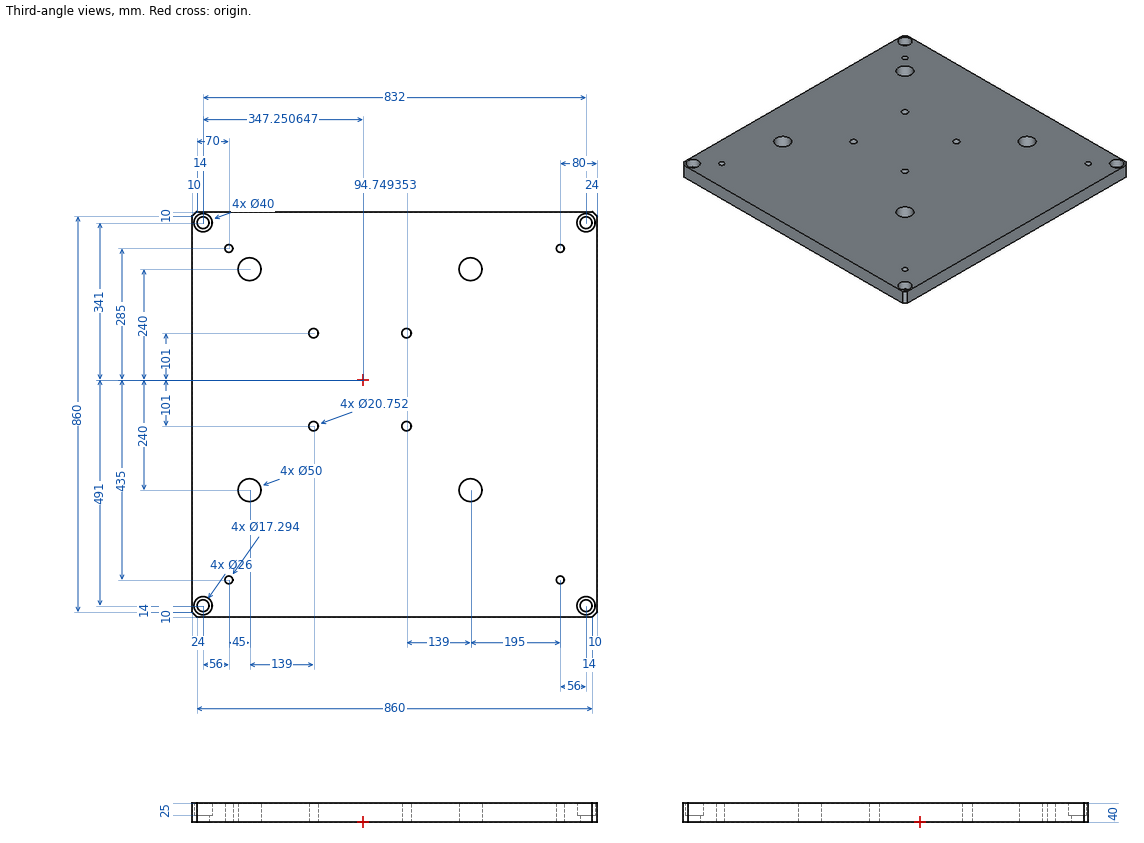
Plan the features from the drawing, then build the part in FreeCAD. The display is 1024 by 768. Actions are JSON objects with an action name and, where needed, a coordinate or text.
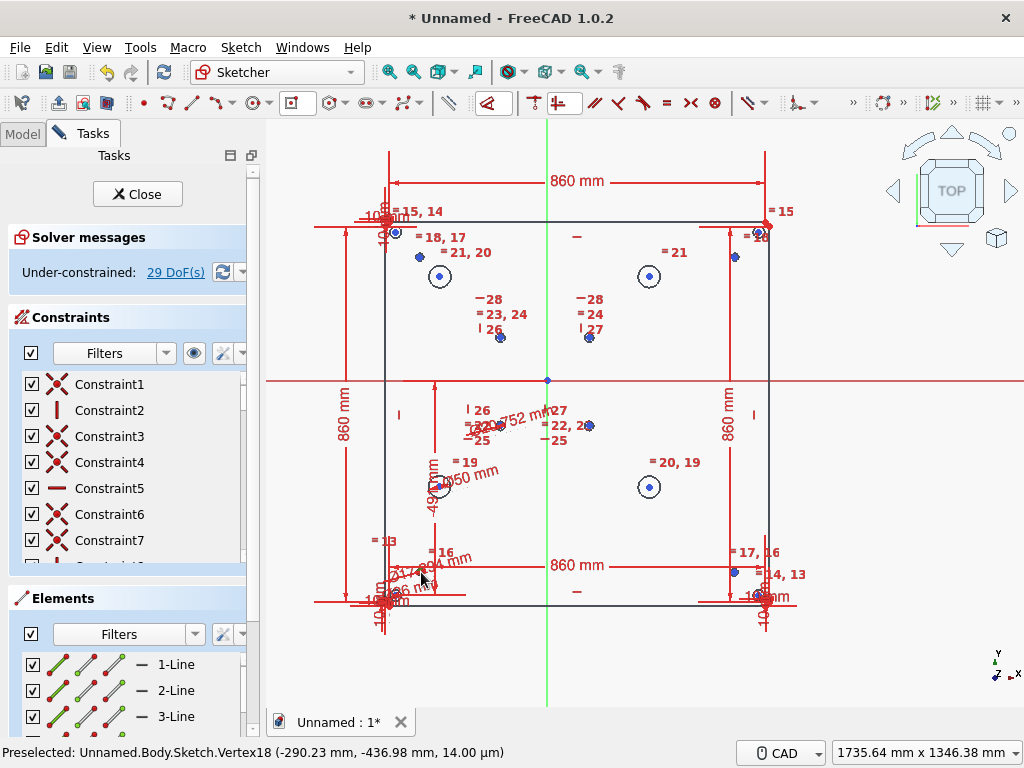
{"action": "key", "text": "i"}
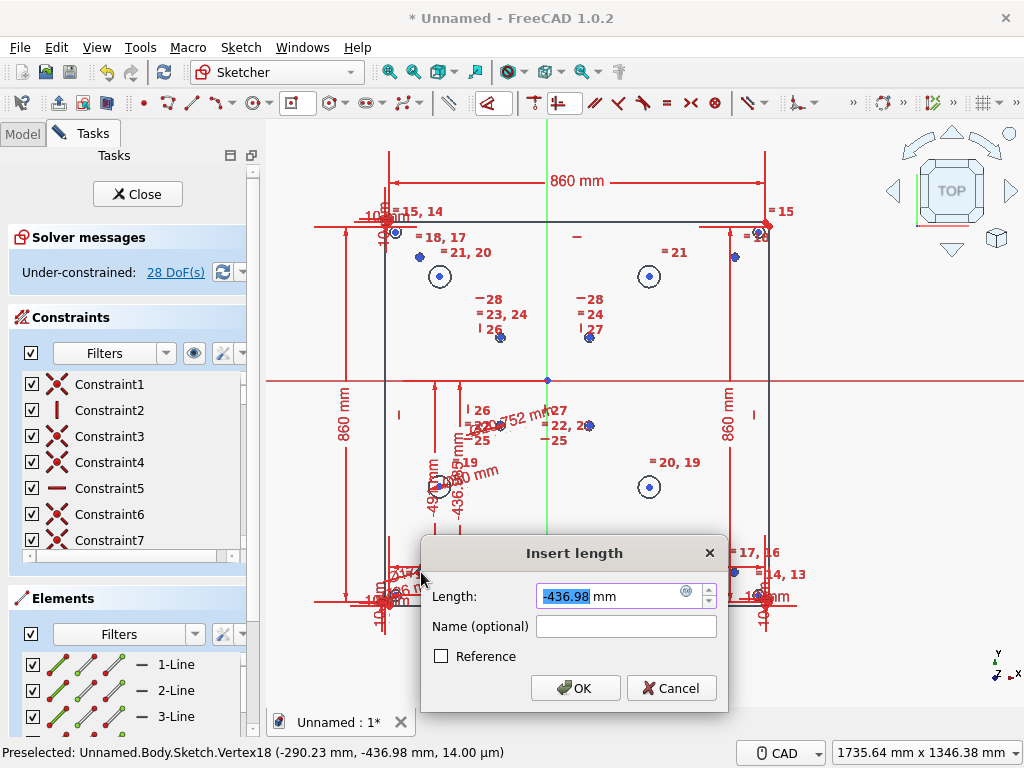
{"action": "type", "text": "-435"}
{"action": "key", "text": "Return"}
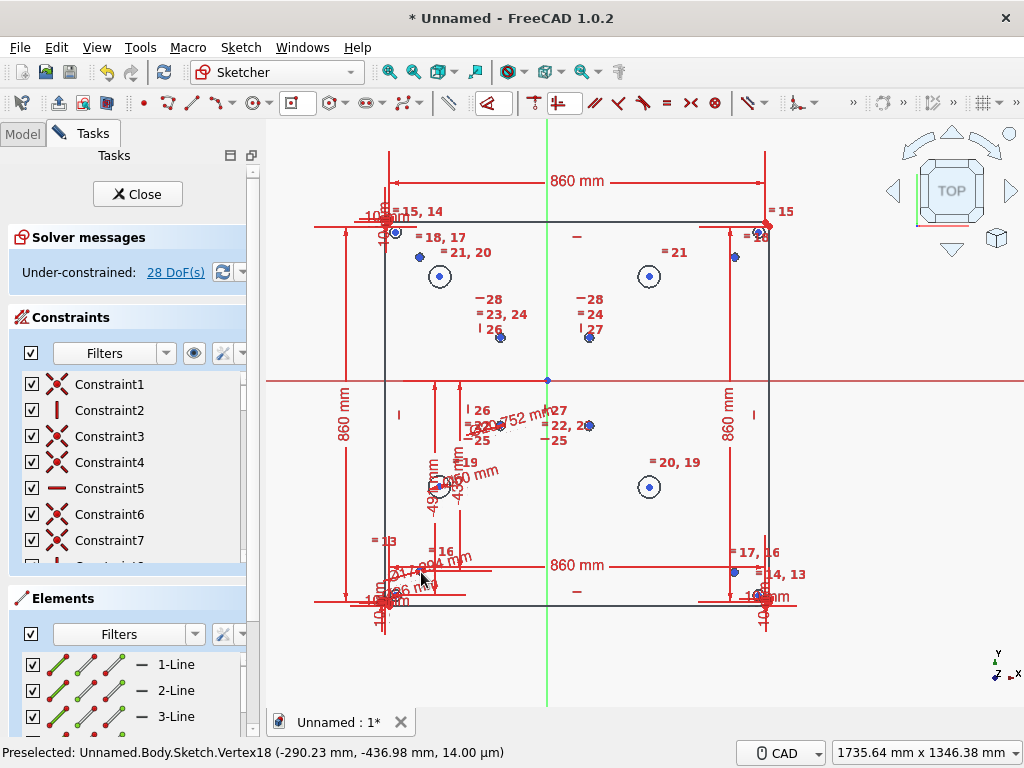
{"action": "left_click", "coordinate": [440, 487]}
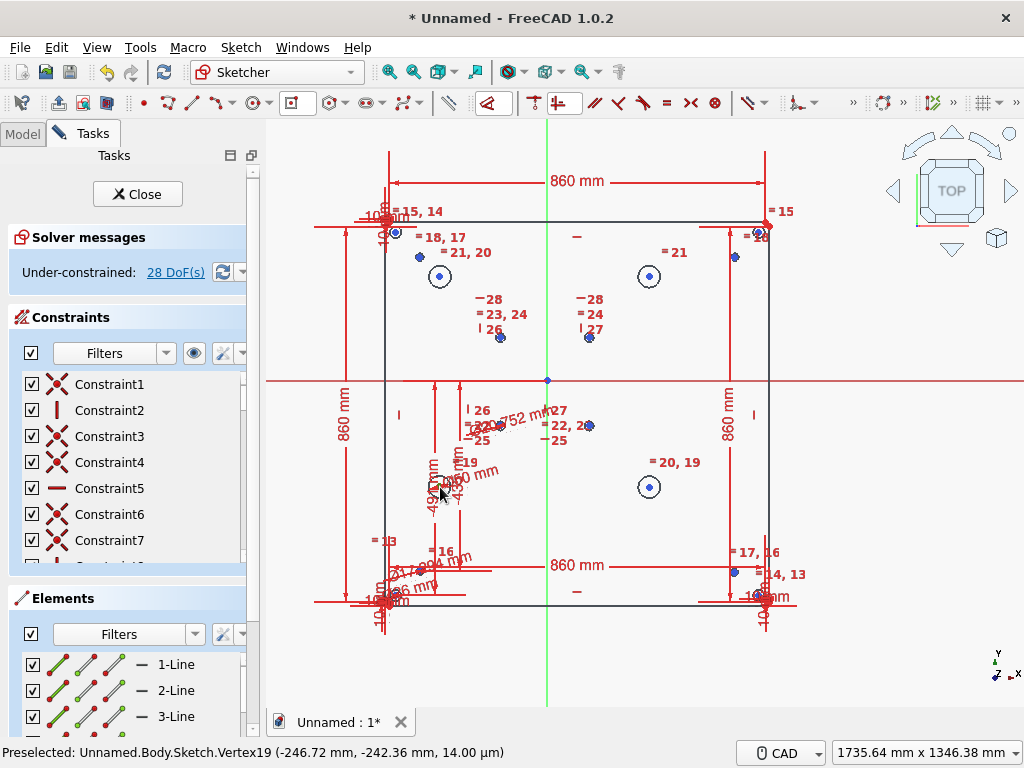
{"action": "key", "text": "i"}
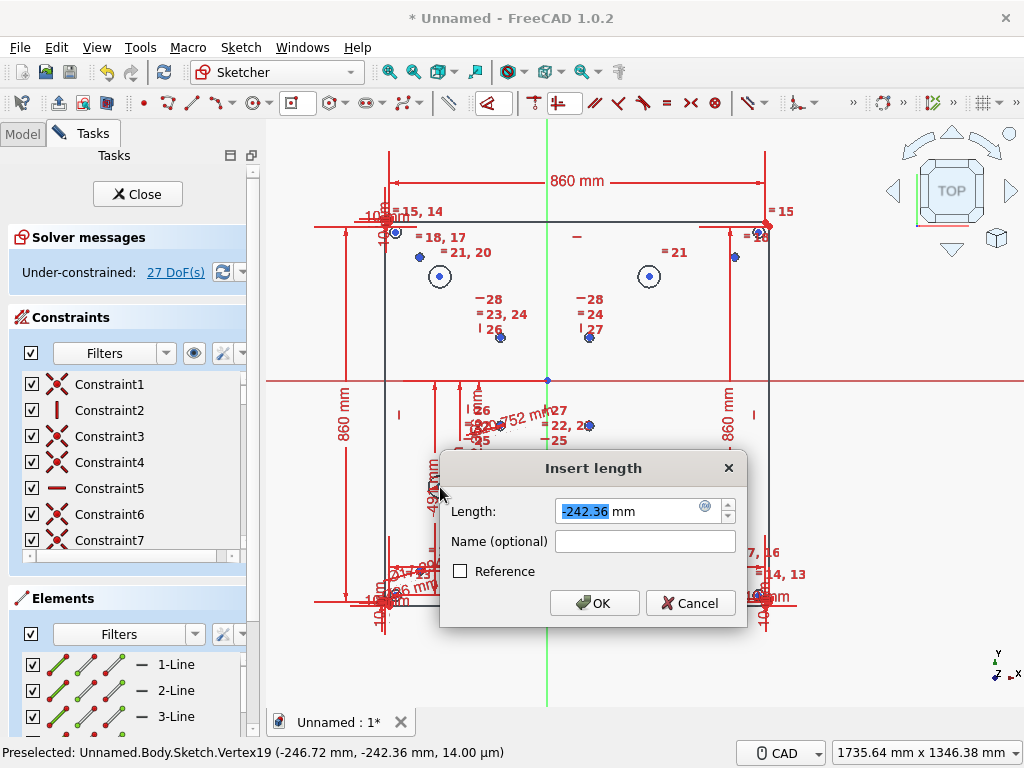
{"action": "type", "text": "-240"}
{"action": "key", "text": "Return"}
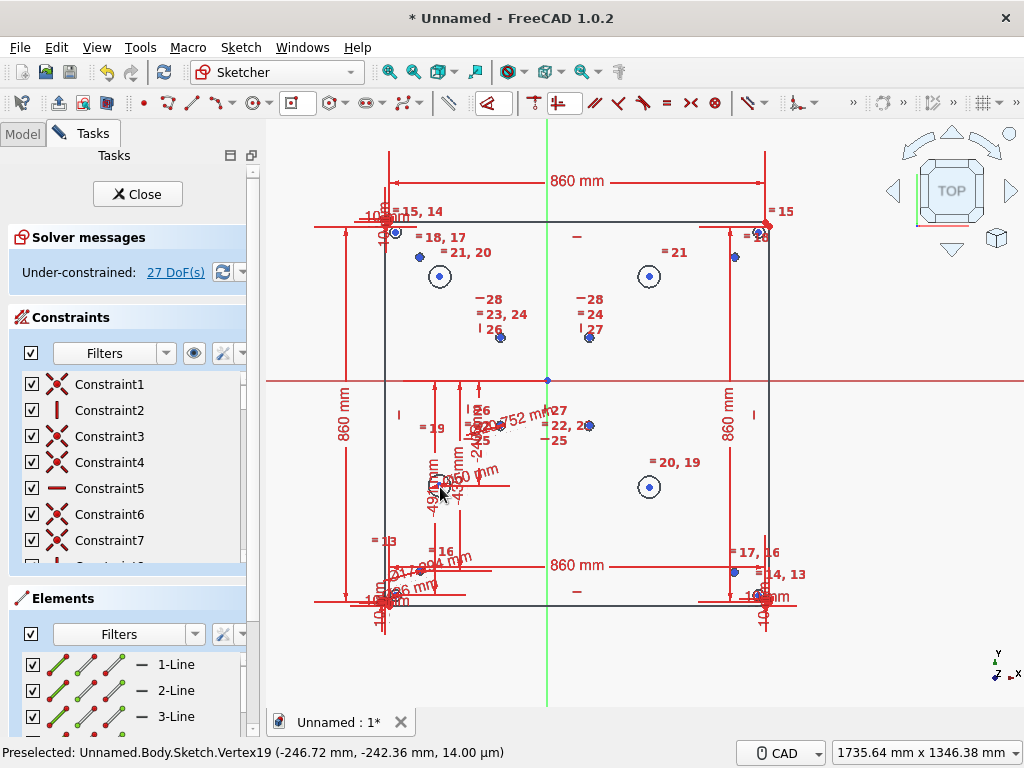
{"action": "left_click", "coordinate": [500, 426]}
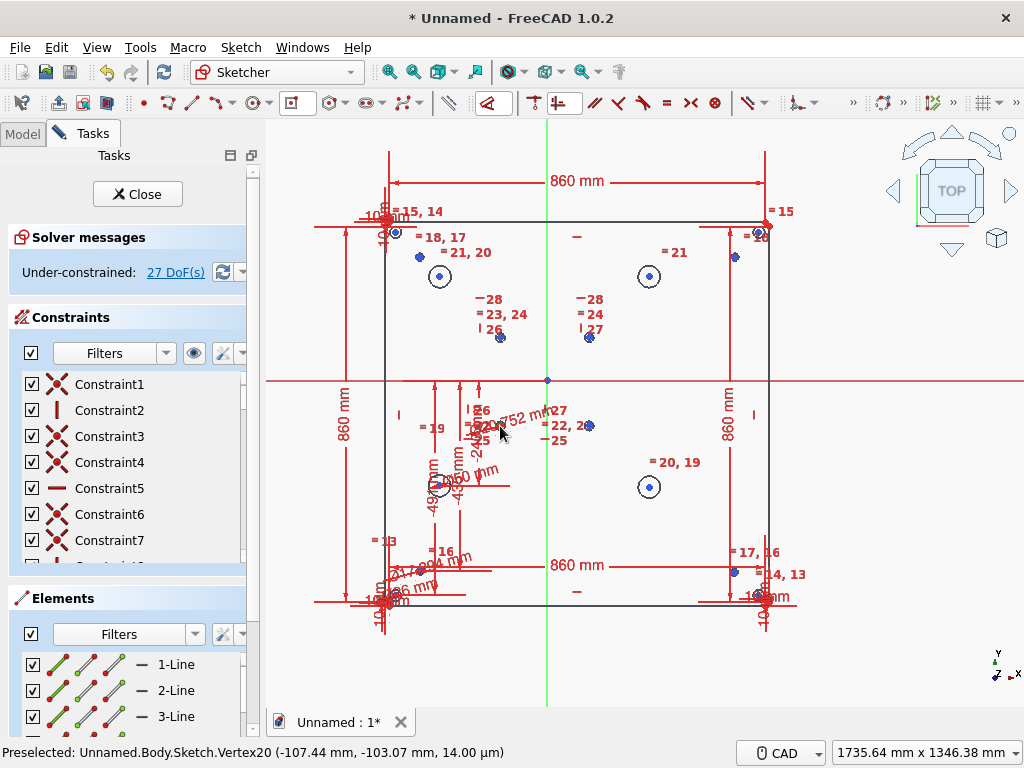
{"action": "key", "text": "i"}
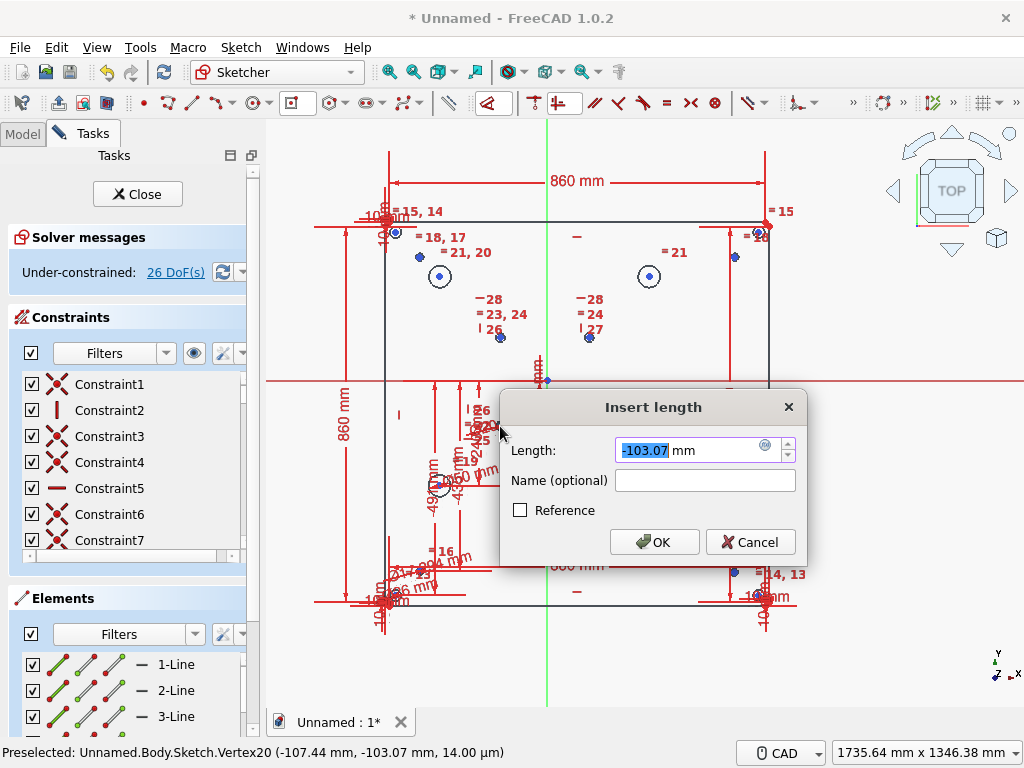
{"action": "type", "text": "-101"}
{"action": "key", "text": "Return"}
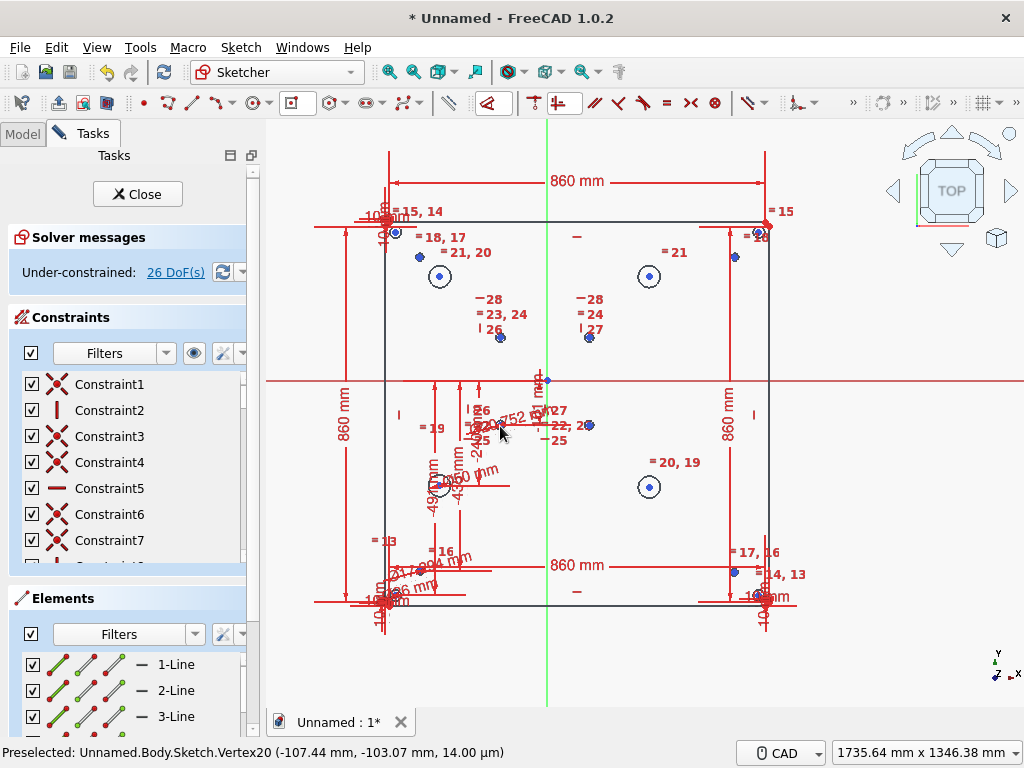
{"action": "left_click", "coordinate": [759, 596]}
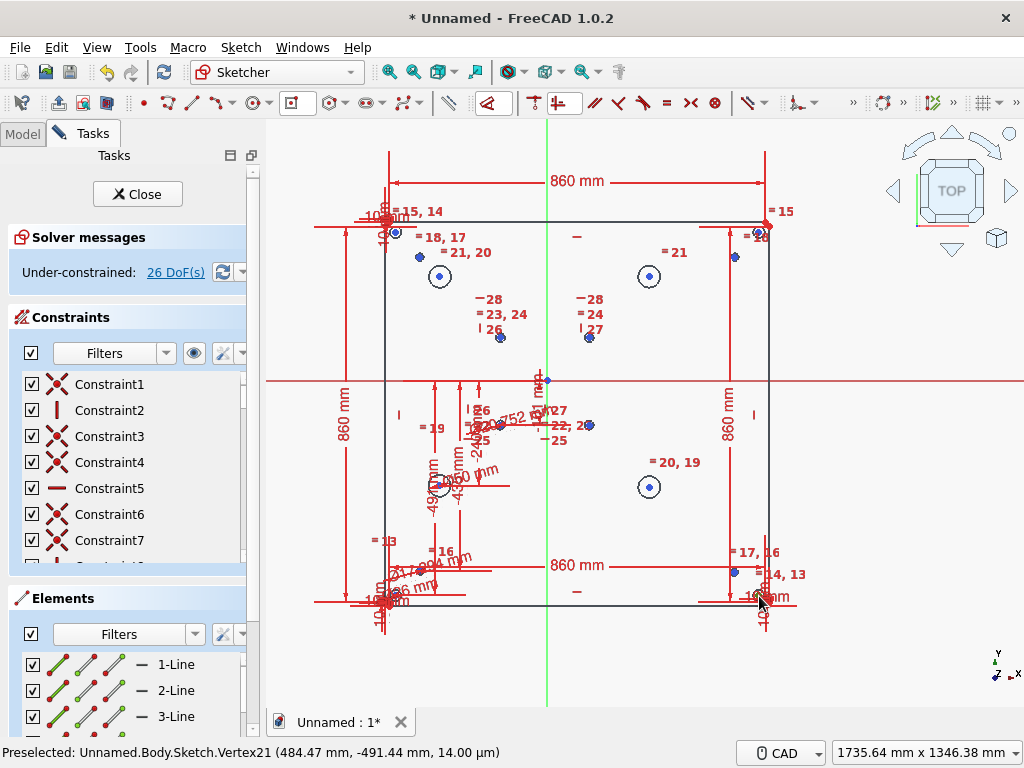
{"action": "key", "text": "i"}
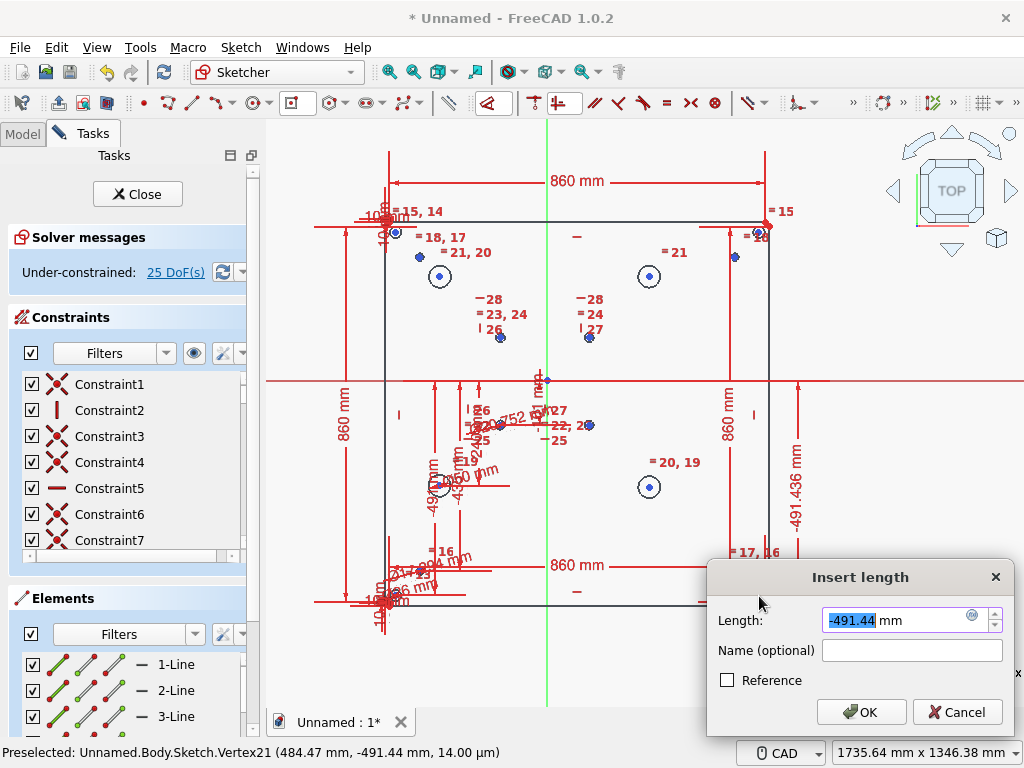
{"action": "type", "text": "-491"}
{"action": "key", "text": "Return"}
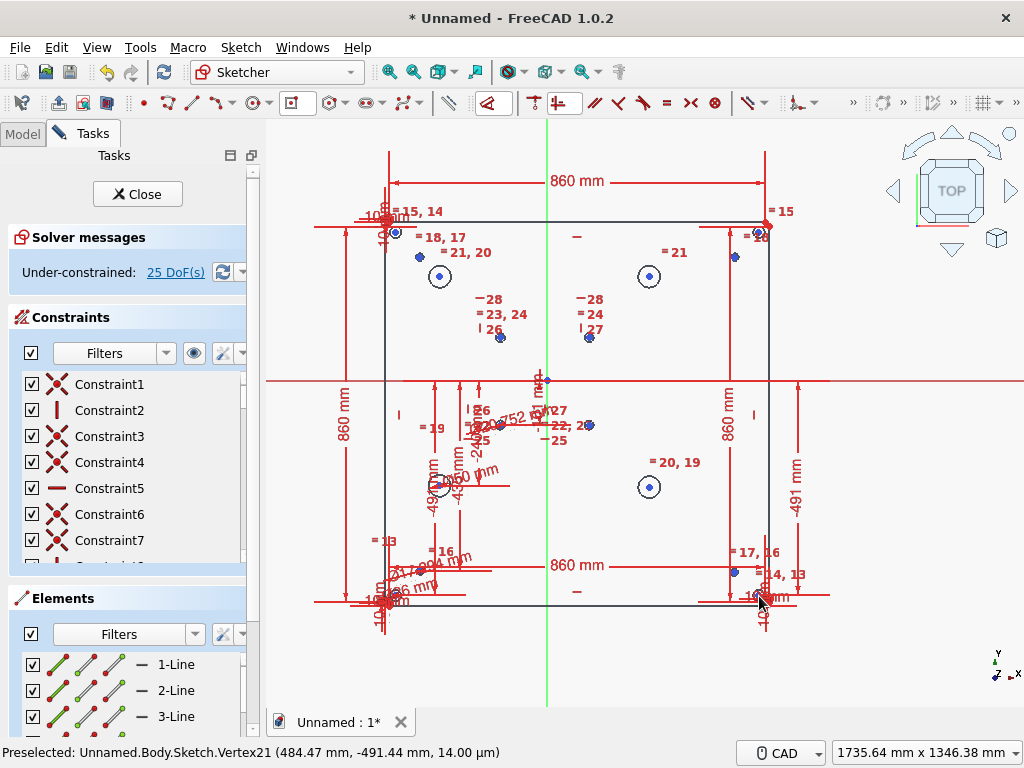
{"action": "left_click", "coordinate": [734, 572]}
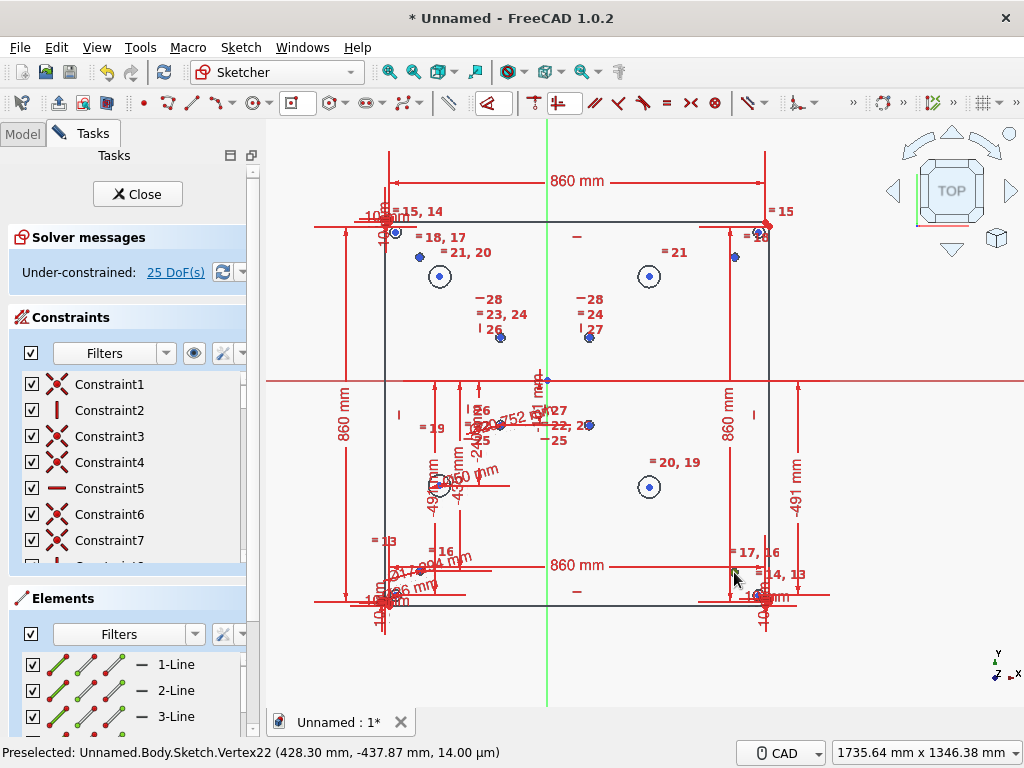
{"action": "key", "text": "i"}